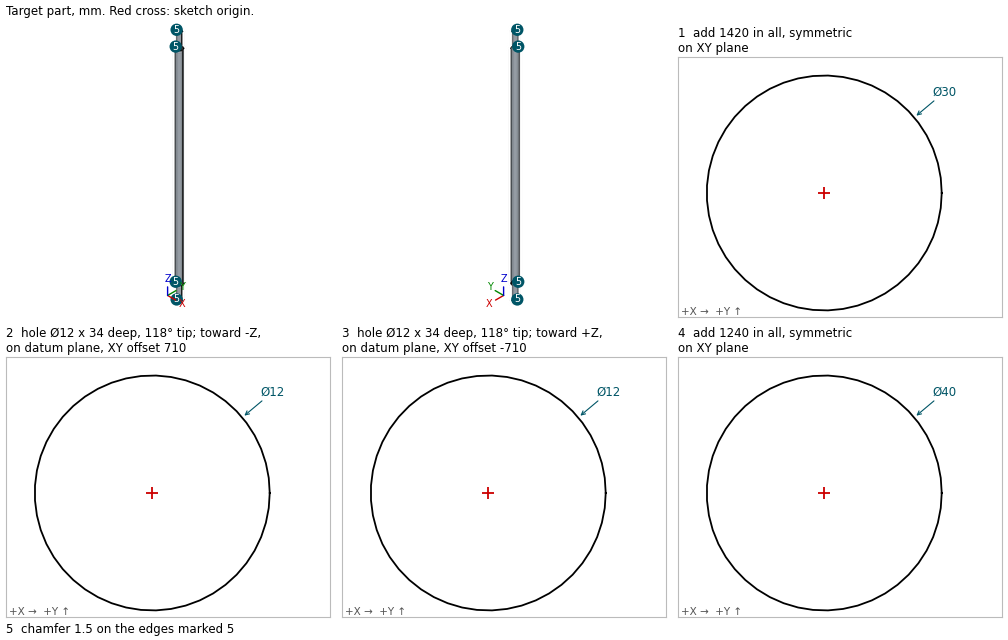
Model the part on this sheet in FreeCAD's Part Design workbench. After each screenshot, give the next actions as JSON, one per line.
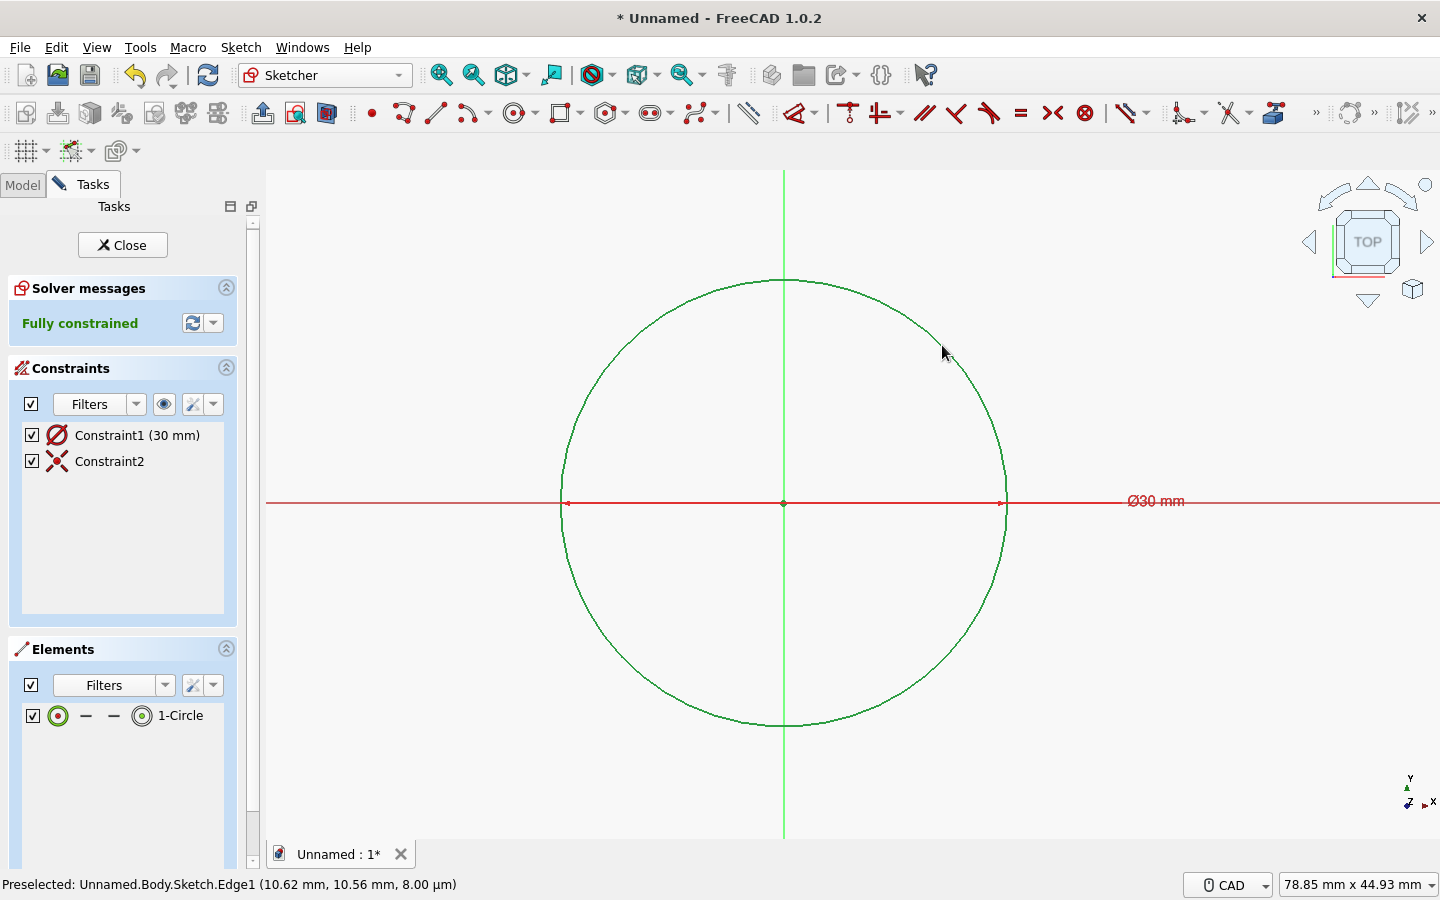
{"action": "left_click", "coordinate": [123, 245]}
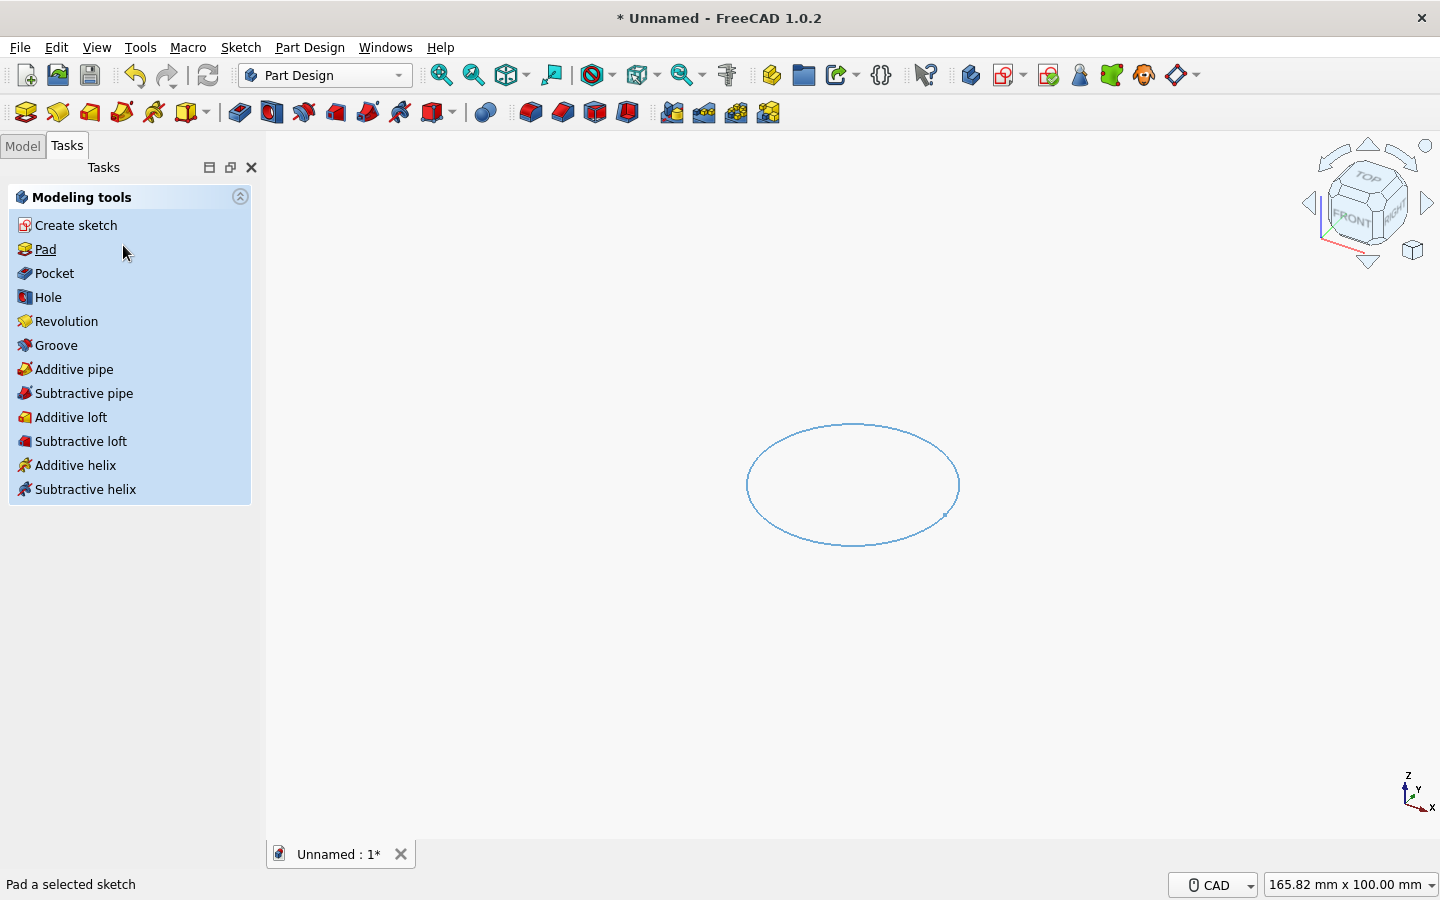
{"action": "left_click", "coordinate": [26, 112]}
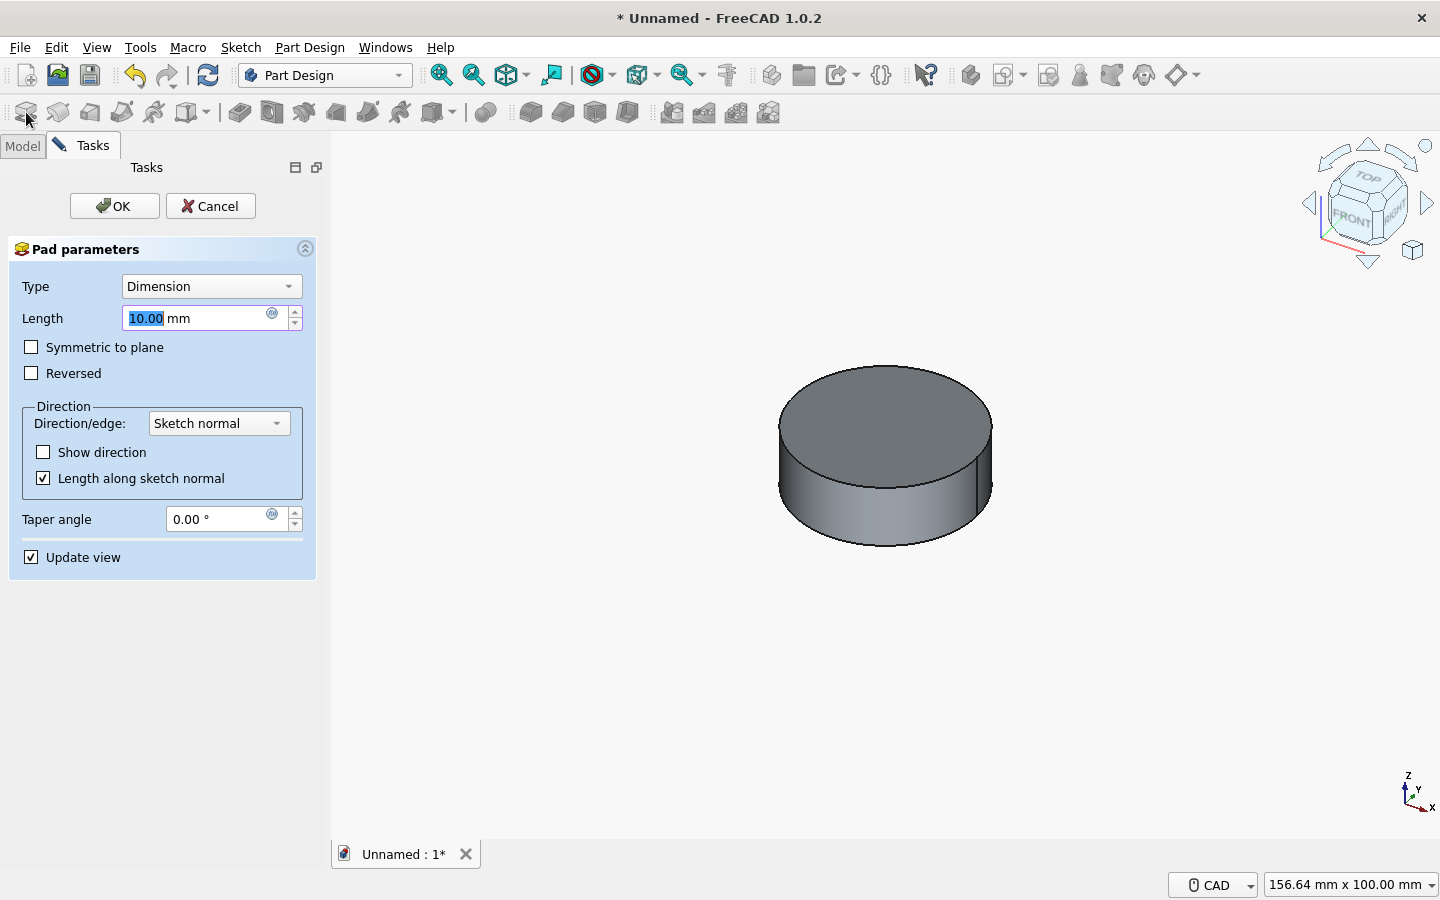
{"action": "type", "text": "1420"}
{"action": "key", "text": "Tab"}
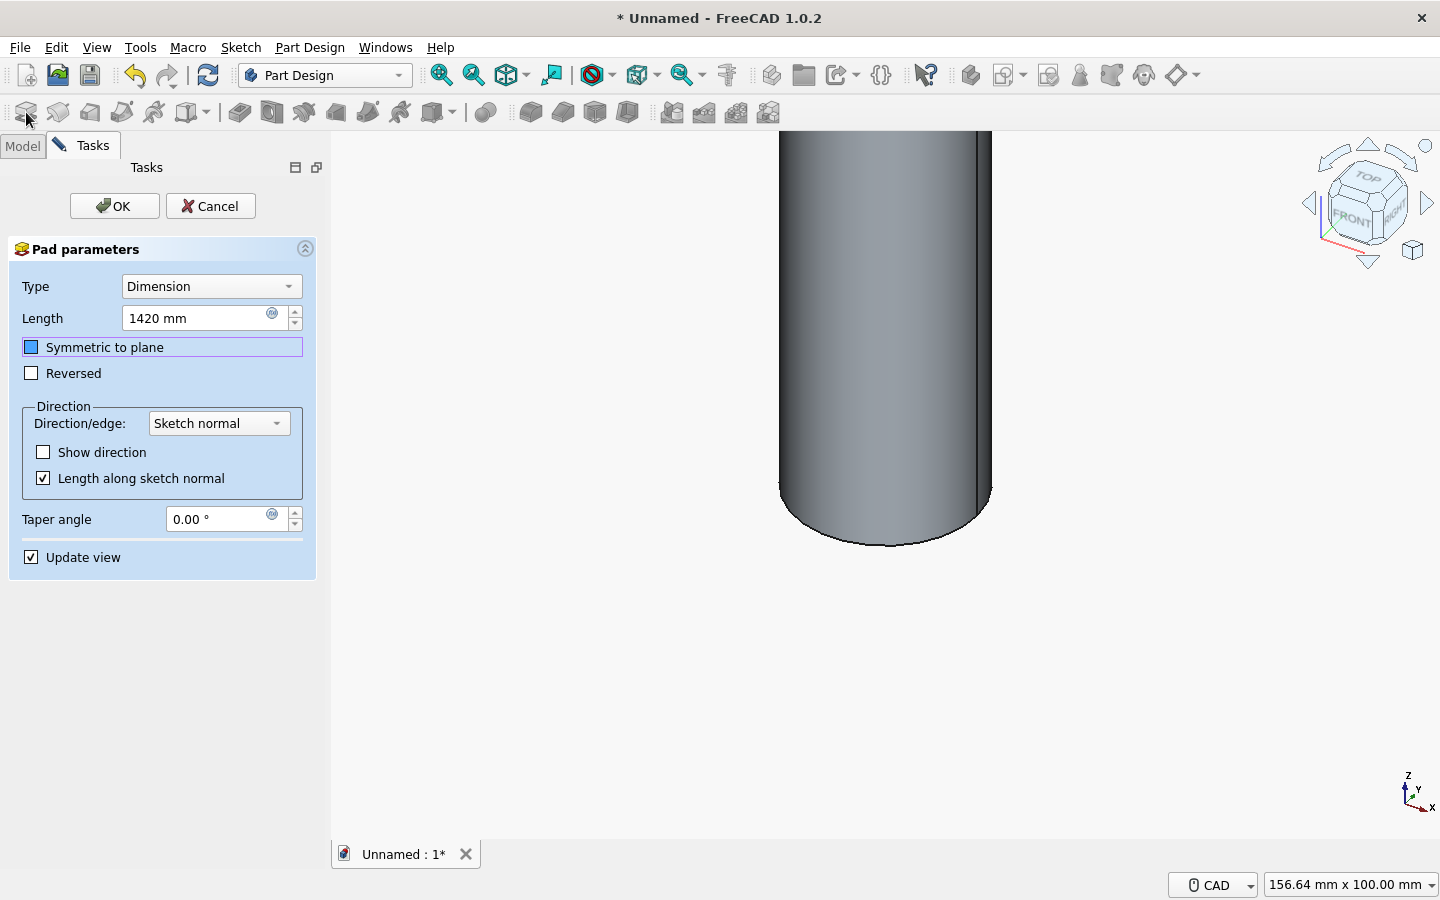
{"action": "left_click", "coordinate": [30, 347]}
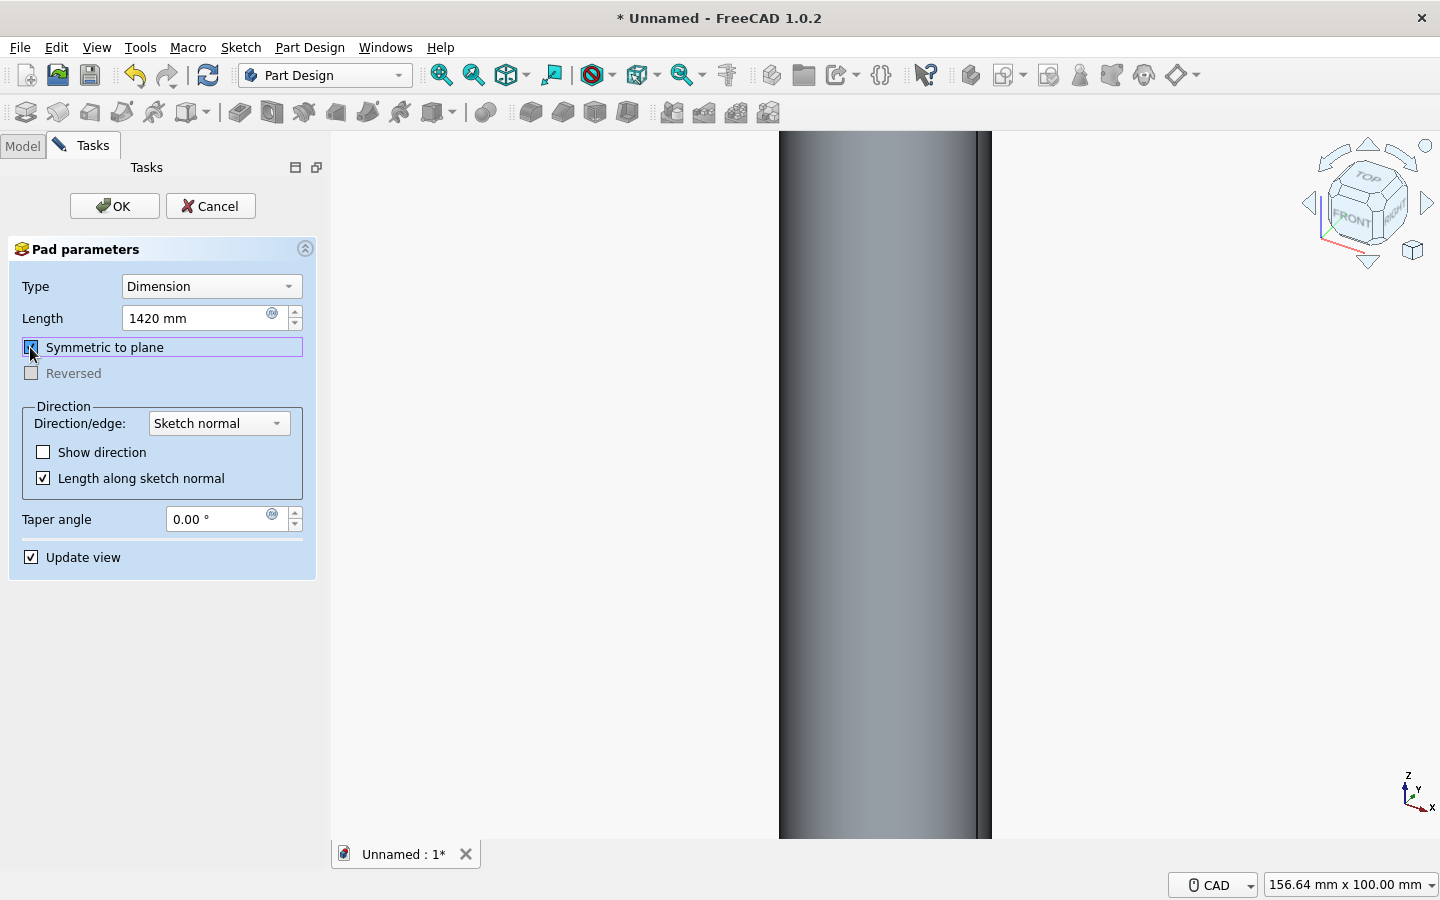
{"action": "left_click", "coordinate": [115, 206]}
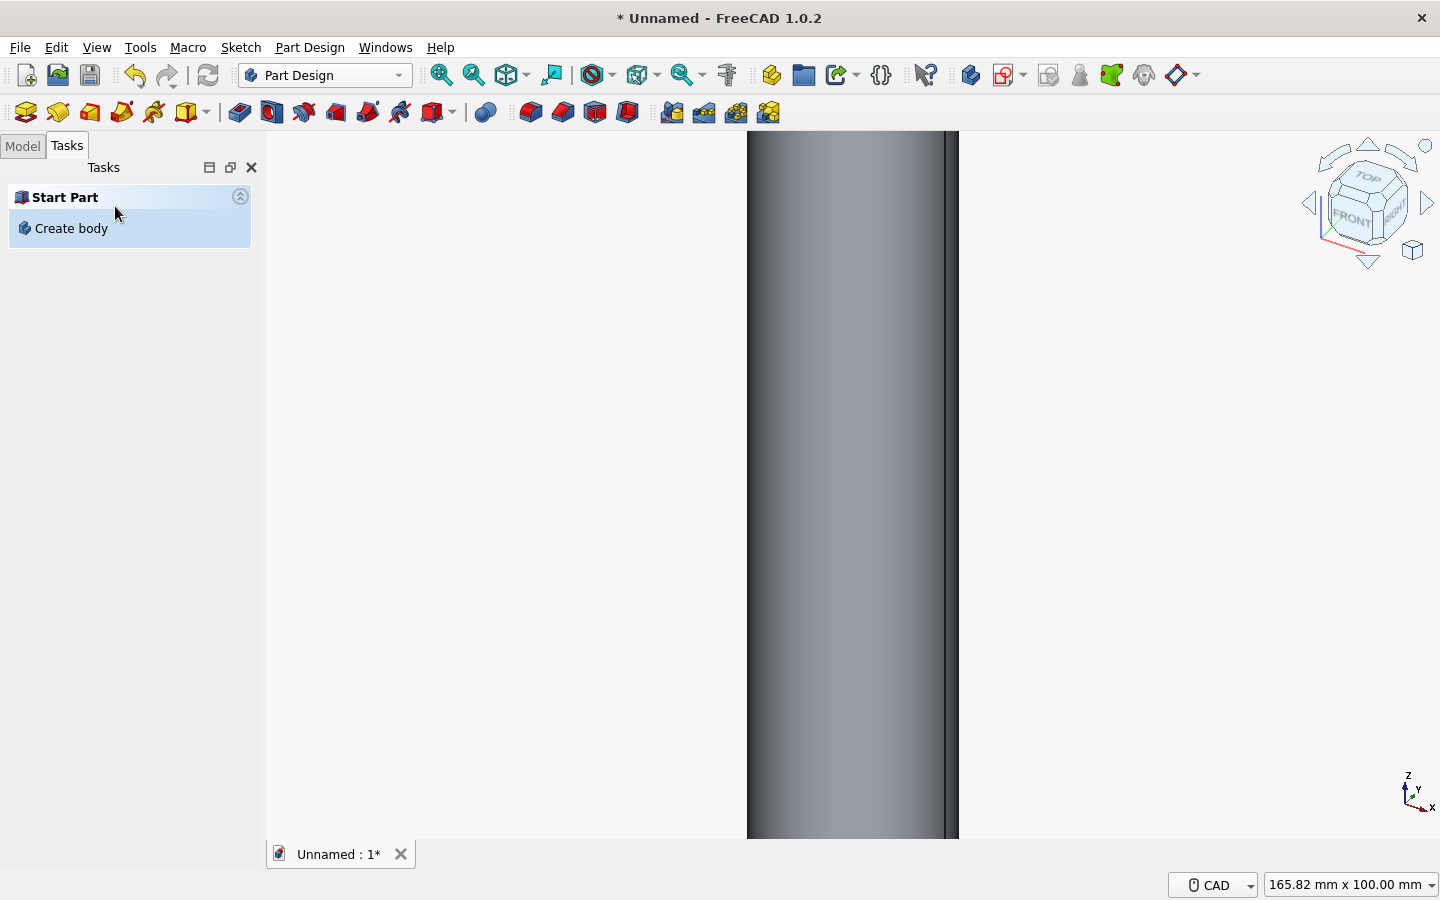
{"action": "left_click", "coordinate": [442, 76]}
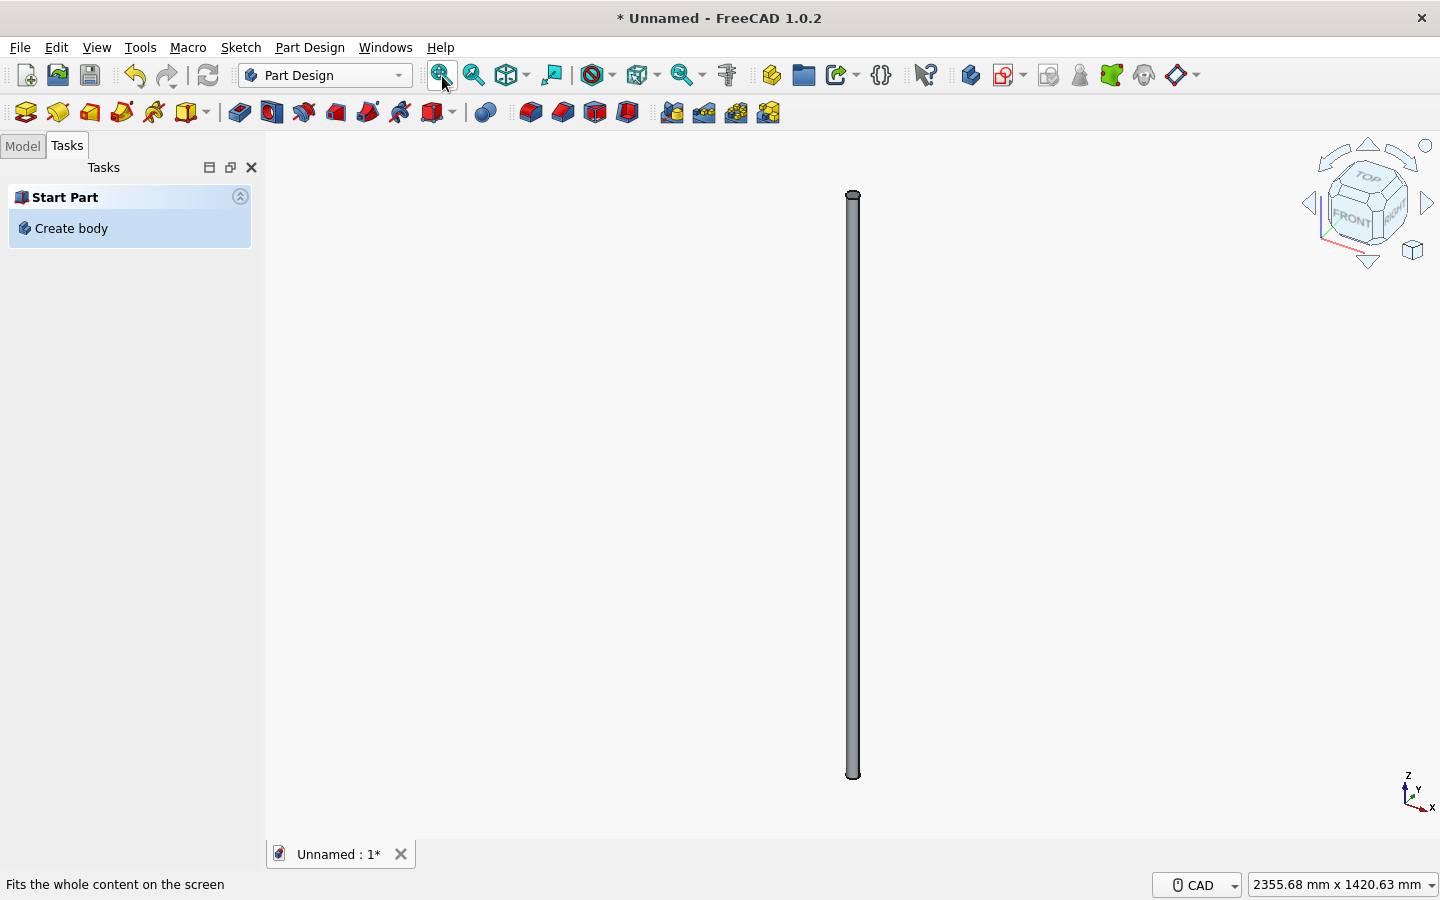
{"action": "key", "text": "0"}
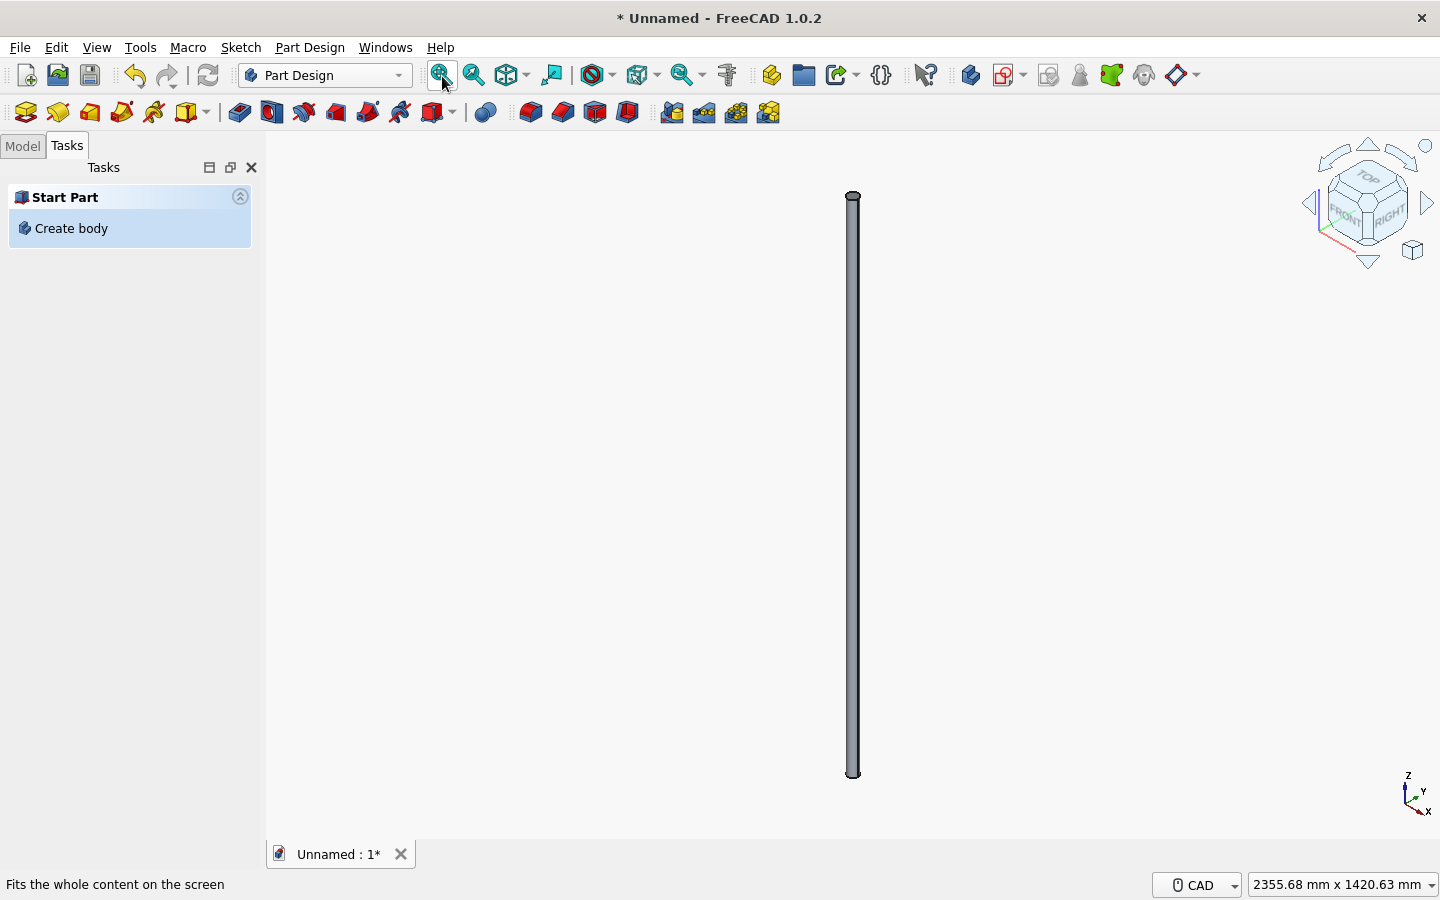
{"action": "key", "text": "2"}